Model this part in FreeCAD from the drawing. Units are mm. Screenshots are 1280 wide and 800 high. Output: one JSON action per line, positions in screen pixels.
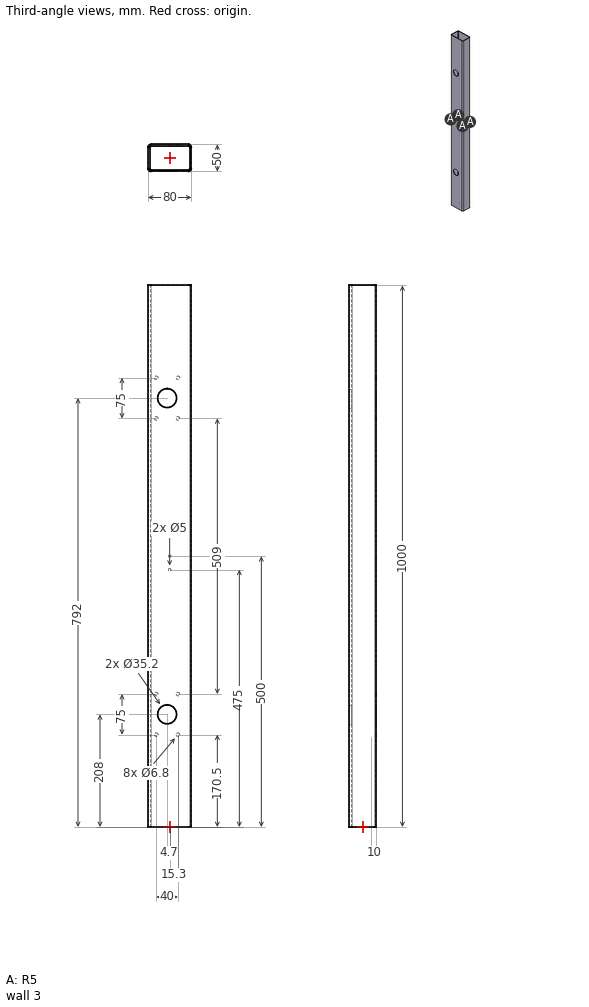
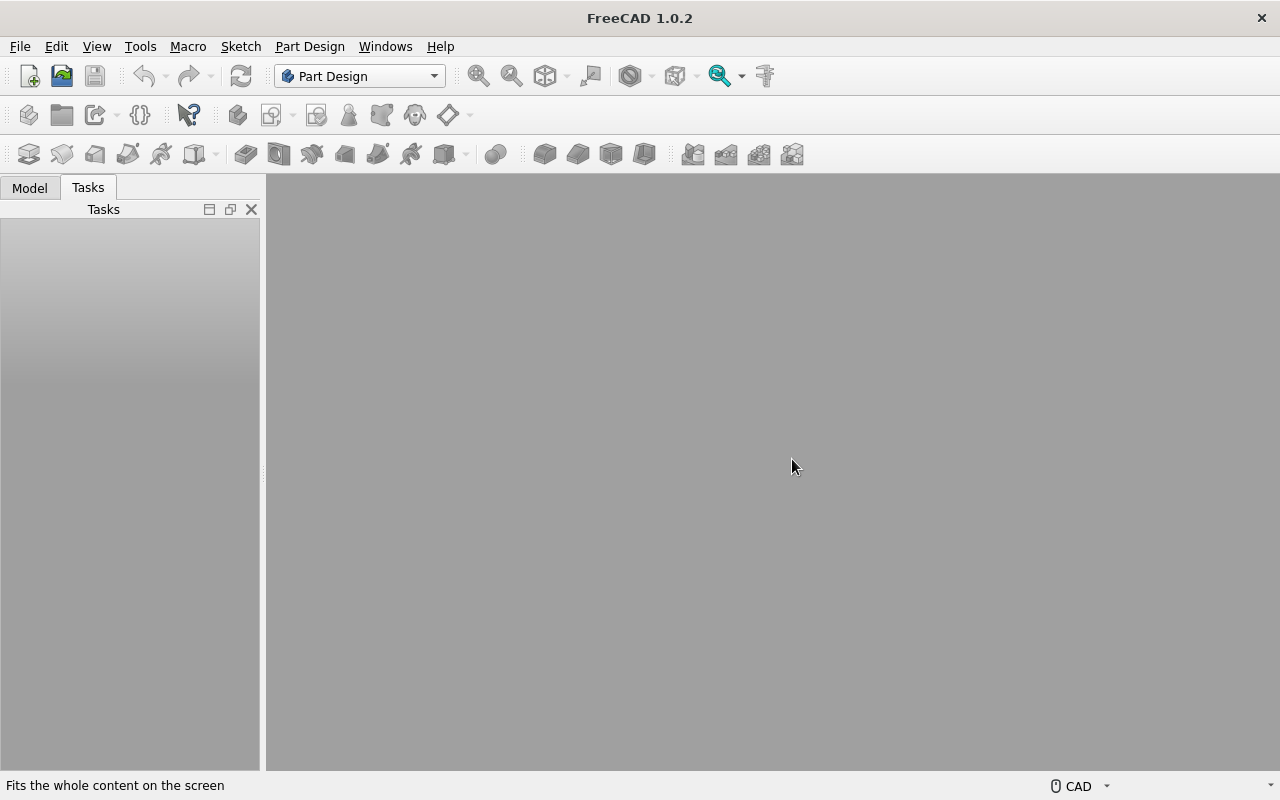
{"action": "left_click", "coordinate": [29, 76]}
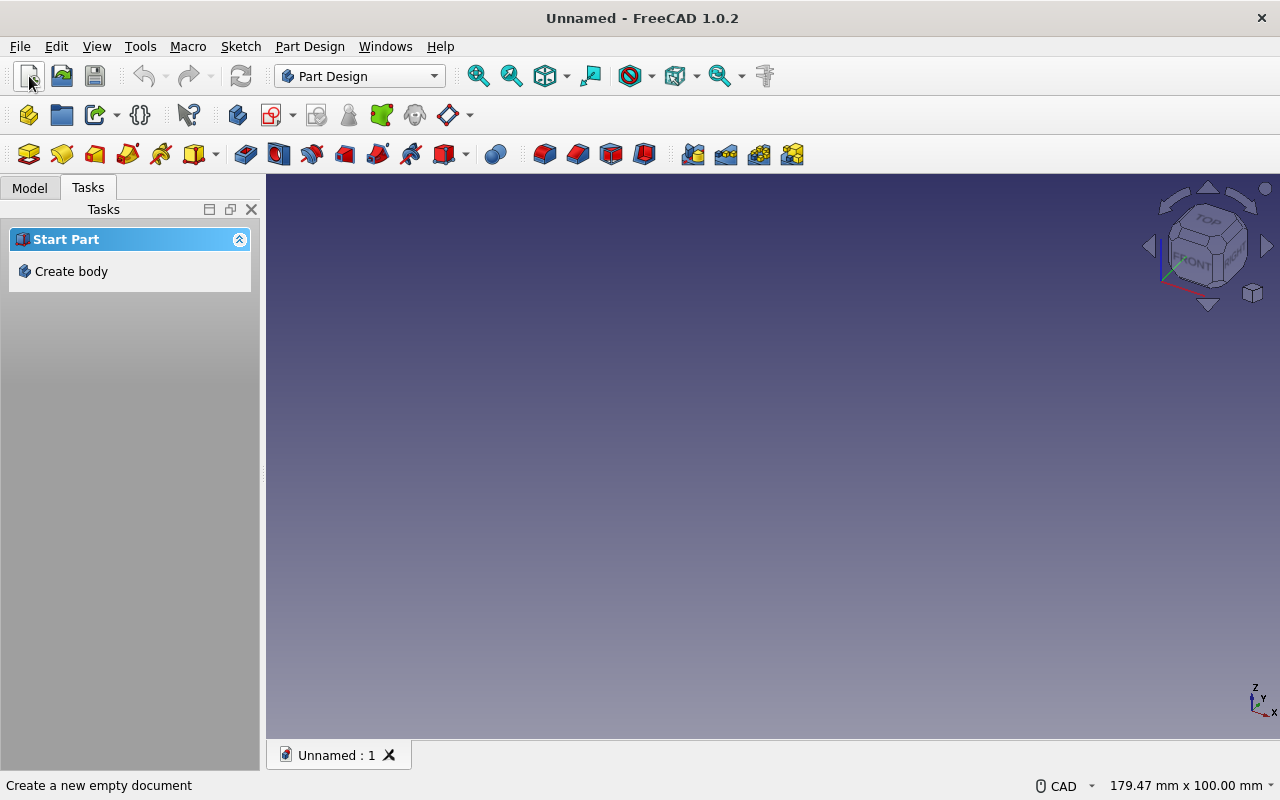
{"action": "left_click", "coordinate": [270, 116]}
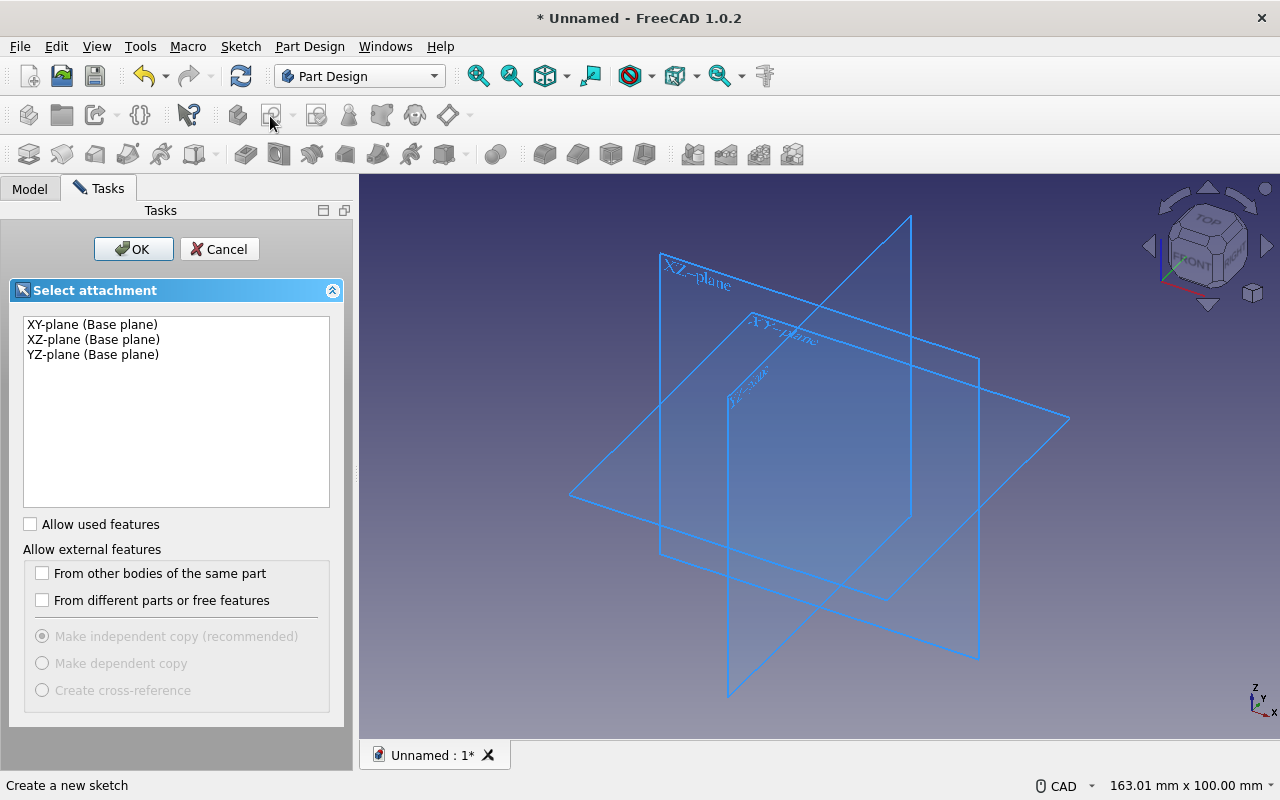
{"action": "left_click", "coordinate": [84, 324]}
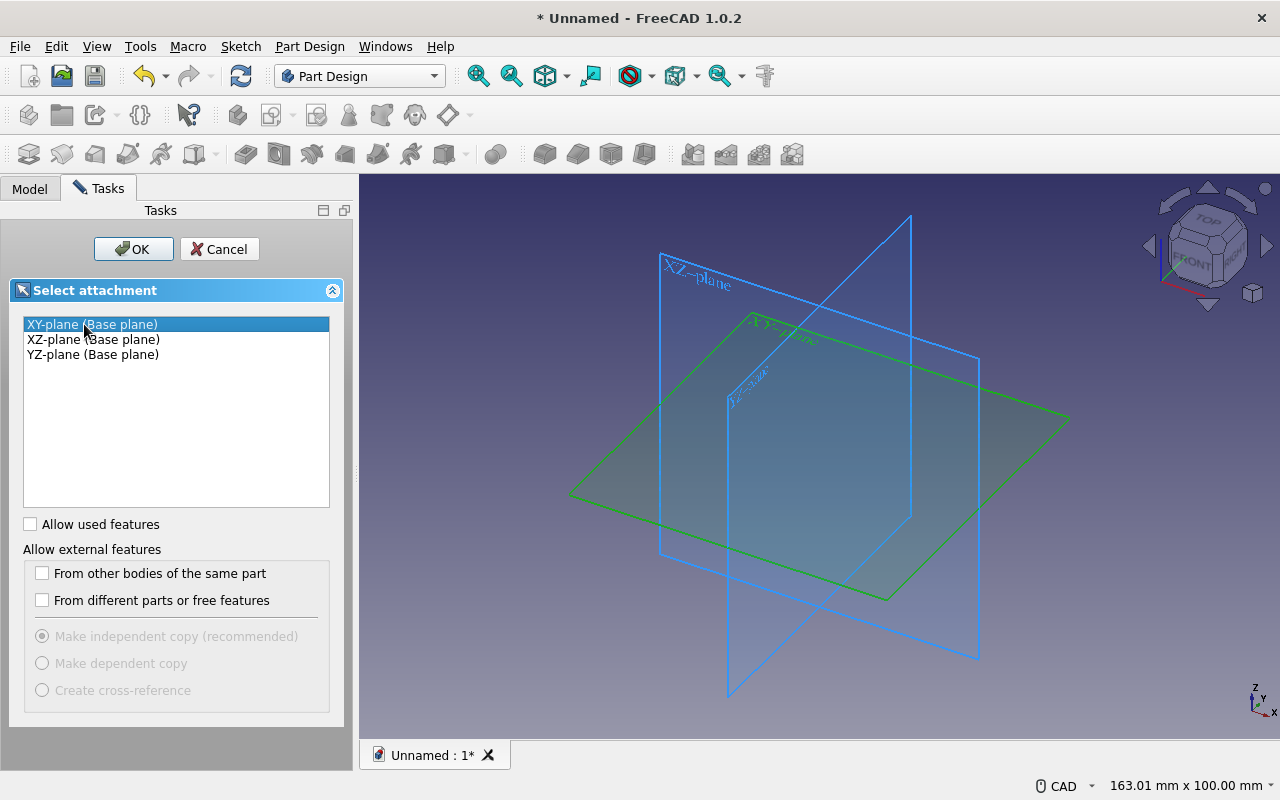
{"action": "left_click", "coordinate": [134, 249]}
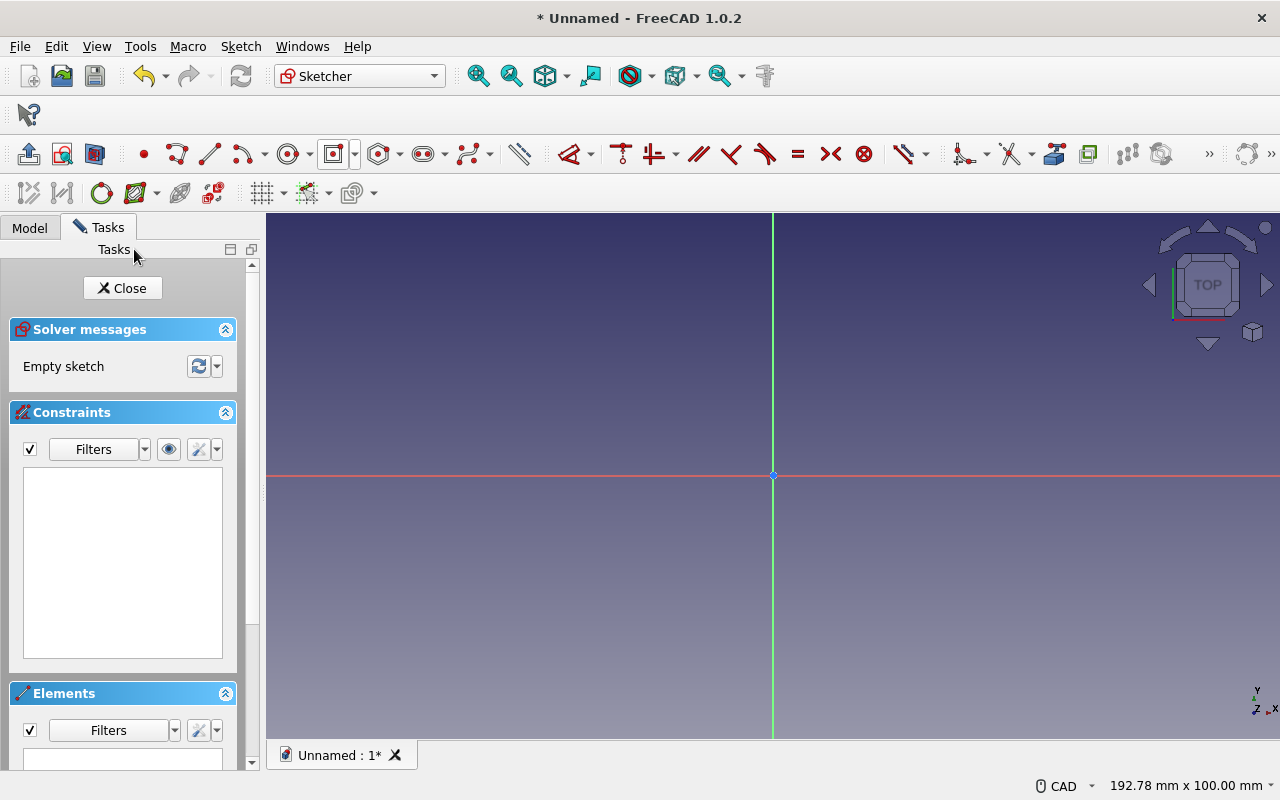
{"action": "left_click", "coordinate": [332, 154]}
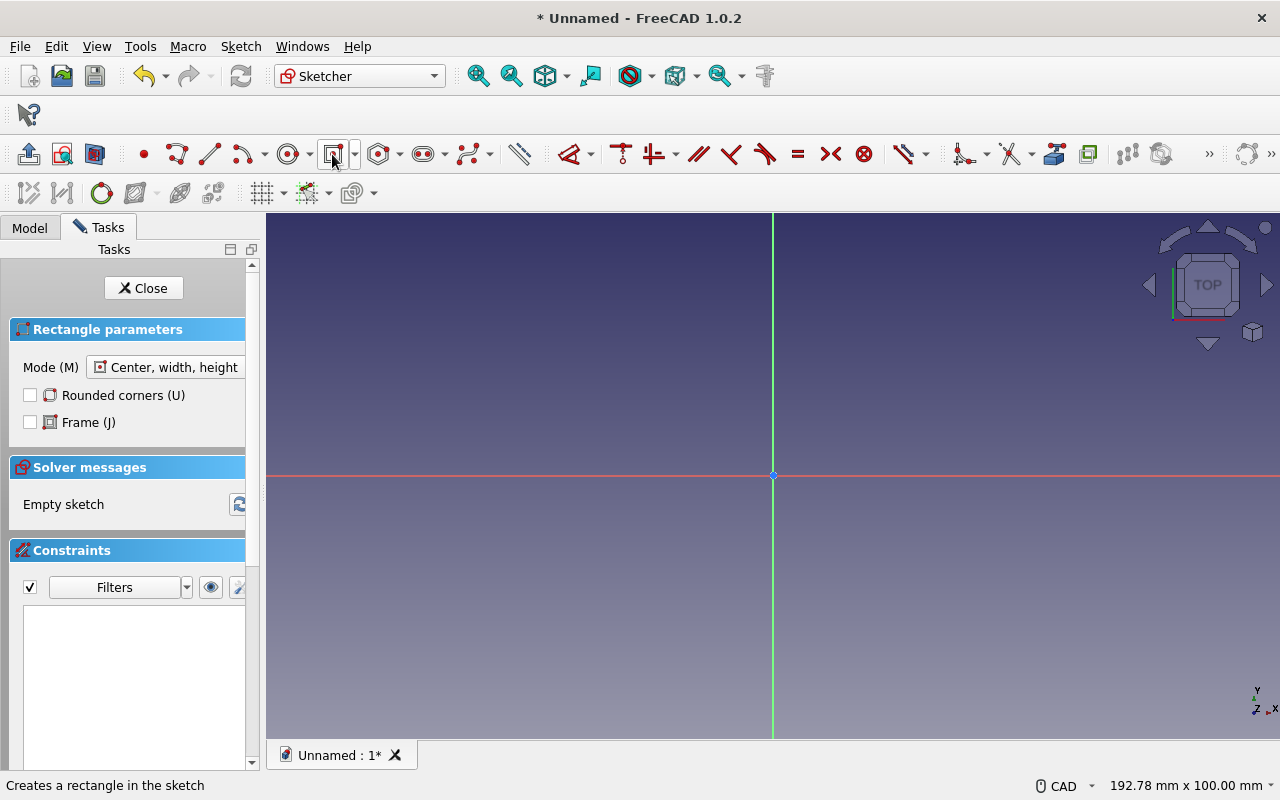
{"action": "left_click", "coordinate": [773, 476]}
{"action": "mouse_move", "coordinate": [983, 344]}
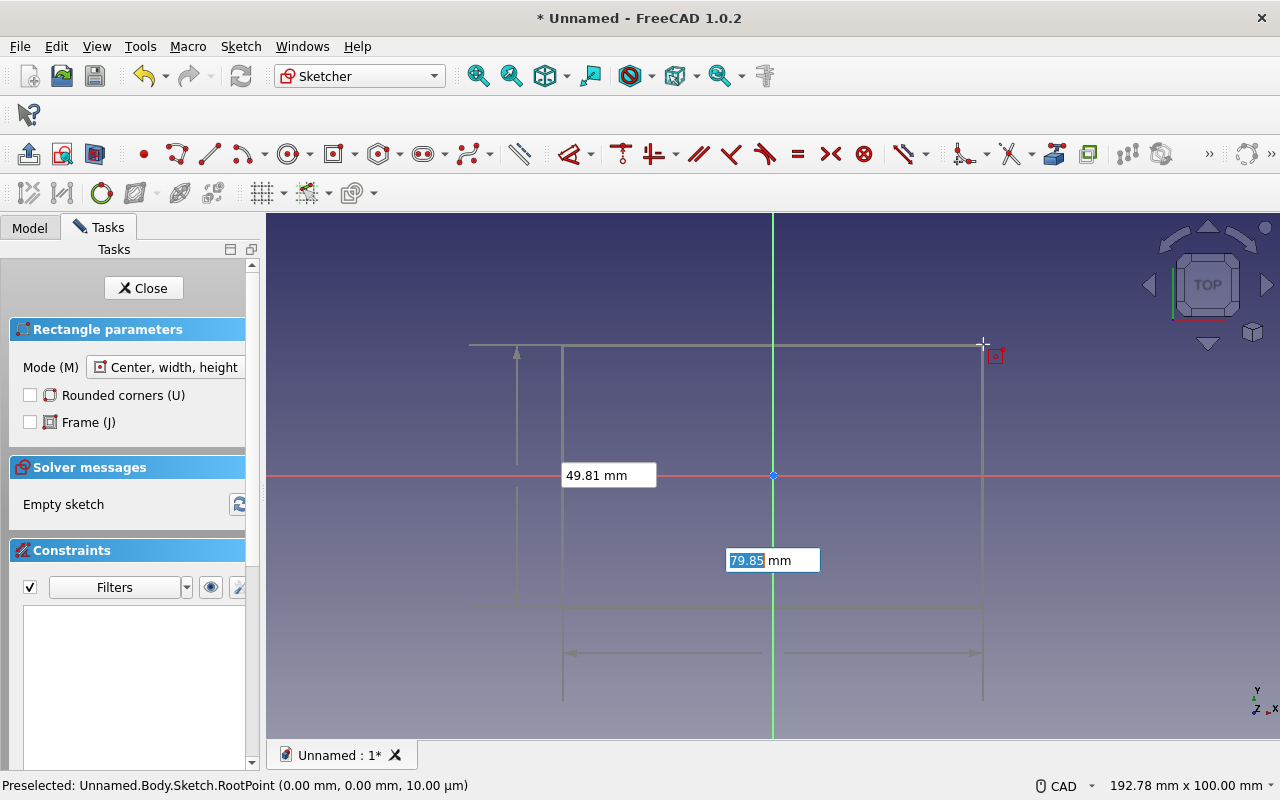
{"action": "type", "text": "80"}
{"action": "key", "text": "Tab"}
{"action": "type", "text": "50"}
{"action": "key", "text": "Return"}
{"action": "key", "text": "Escape"}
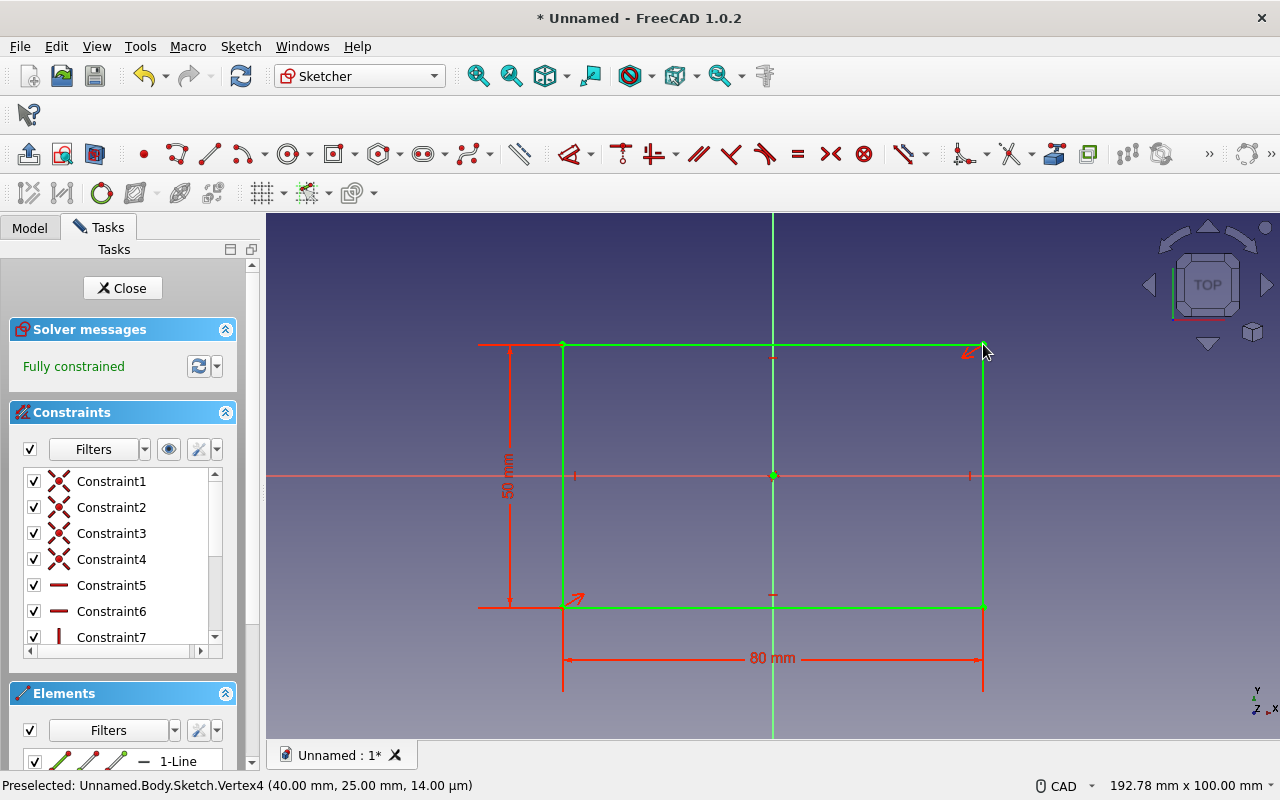
{"action": "left_click", "coordinate": [123, 288]}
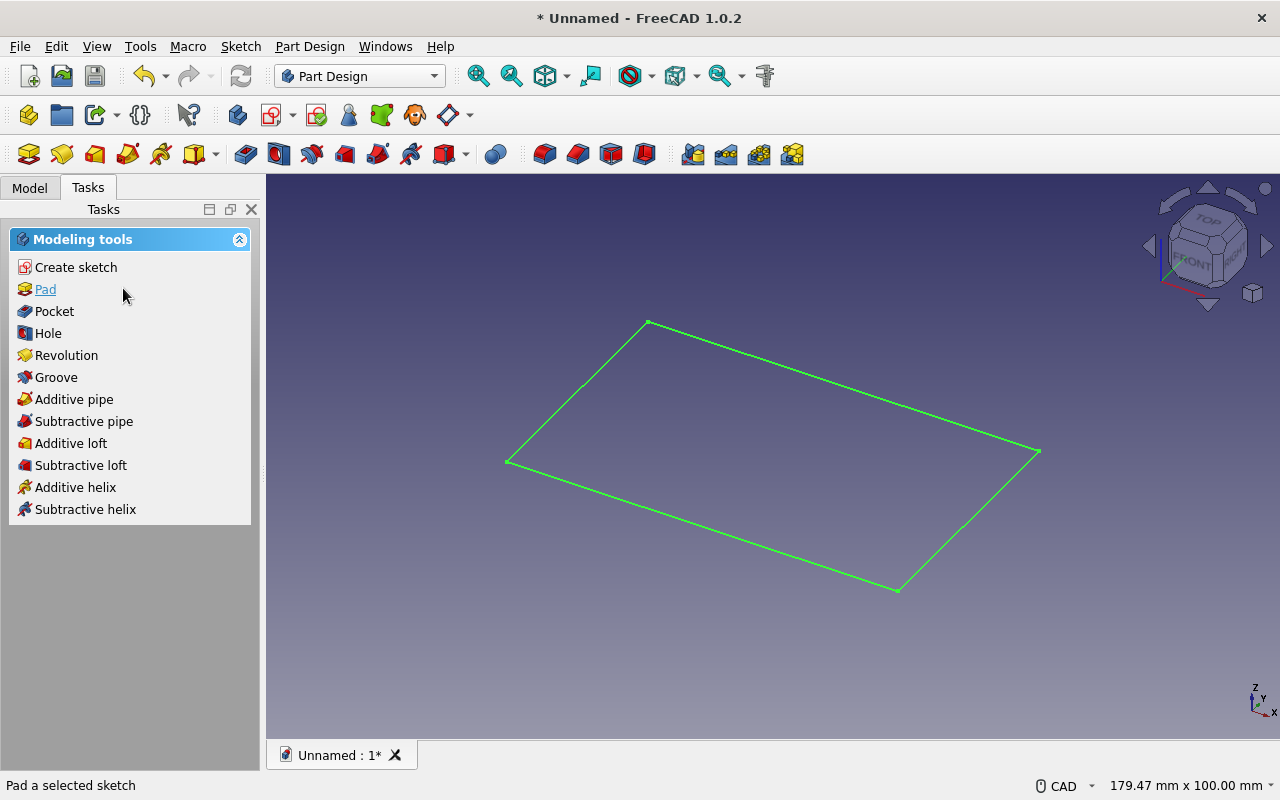
{"action": "left_click", "coordinate": [29, 154]}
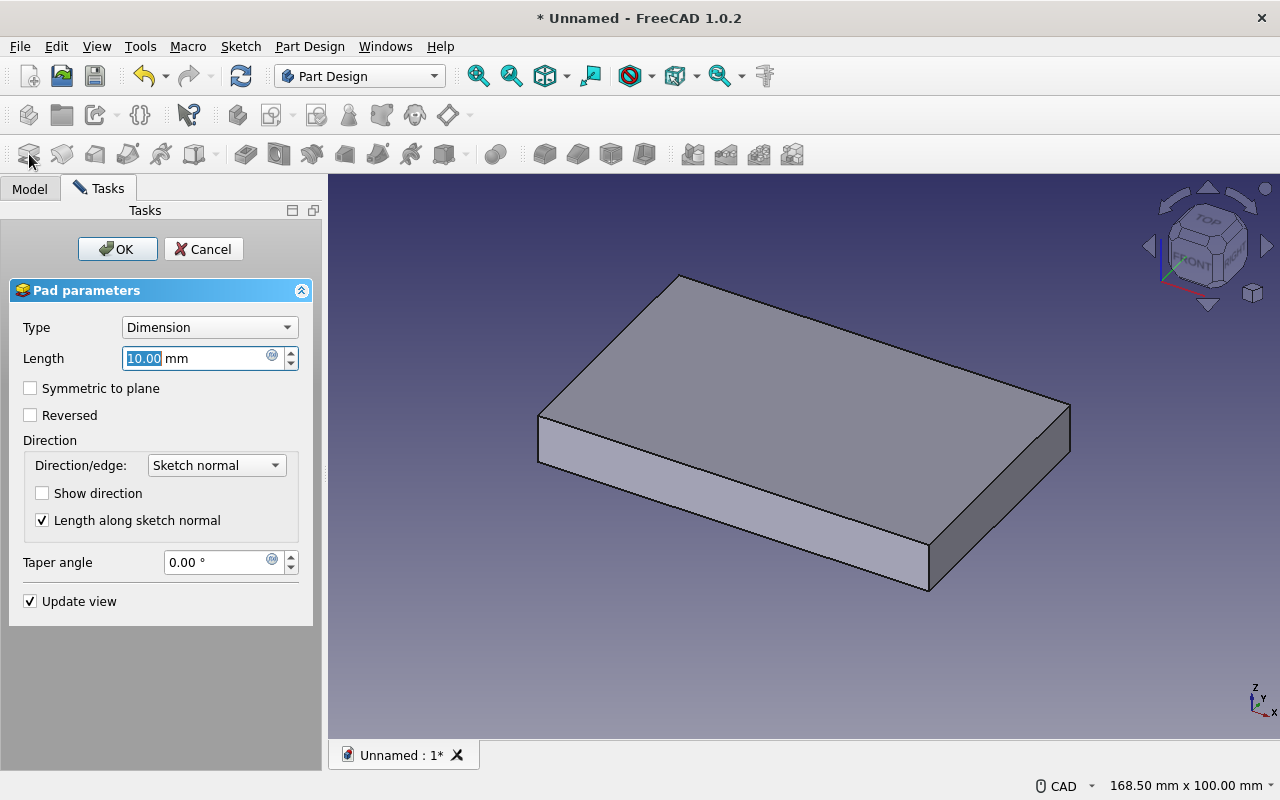
{"action": "type", "text": "1000"}
{"action": "key", "text": "Tab"}